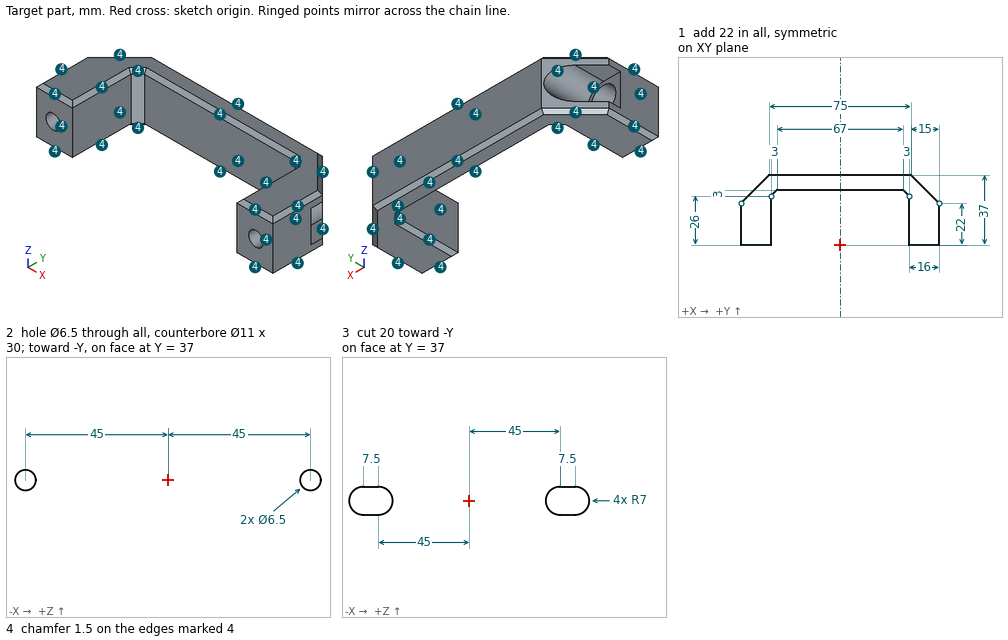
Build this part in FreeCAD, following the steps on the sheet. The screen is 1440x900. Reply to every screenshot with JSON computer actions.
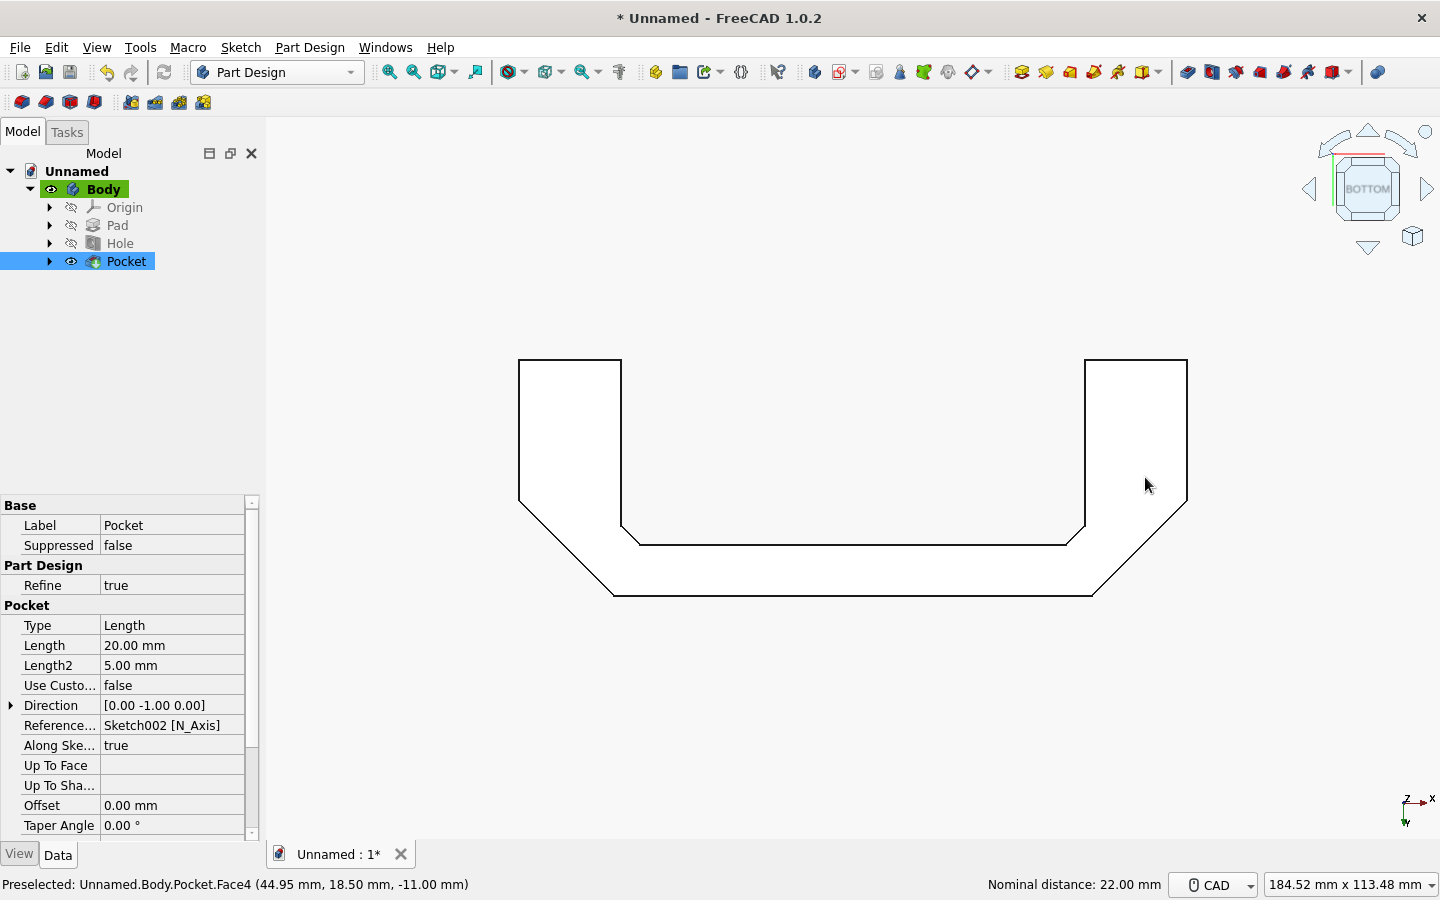
{"action": "left_click", "coordinate": [46, 102]}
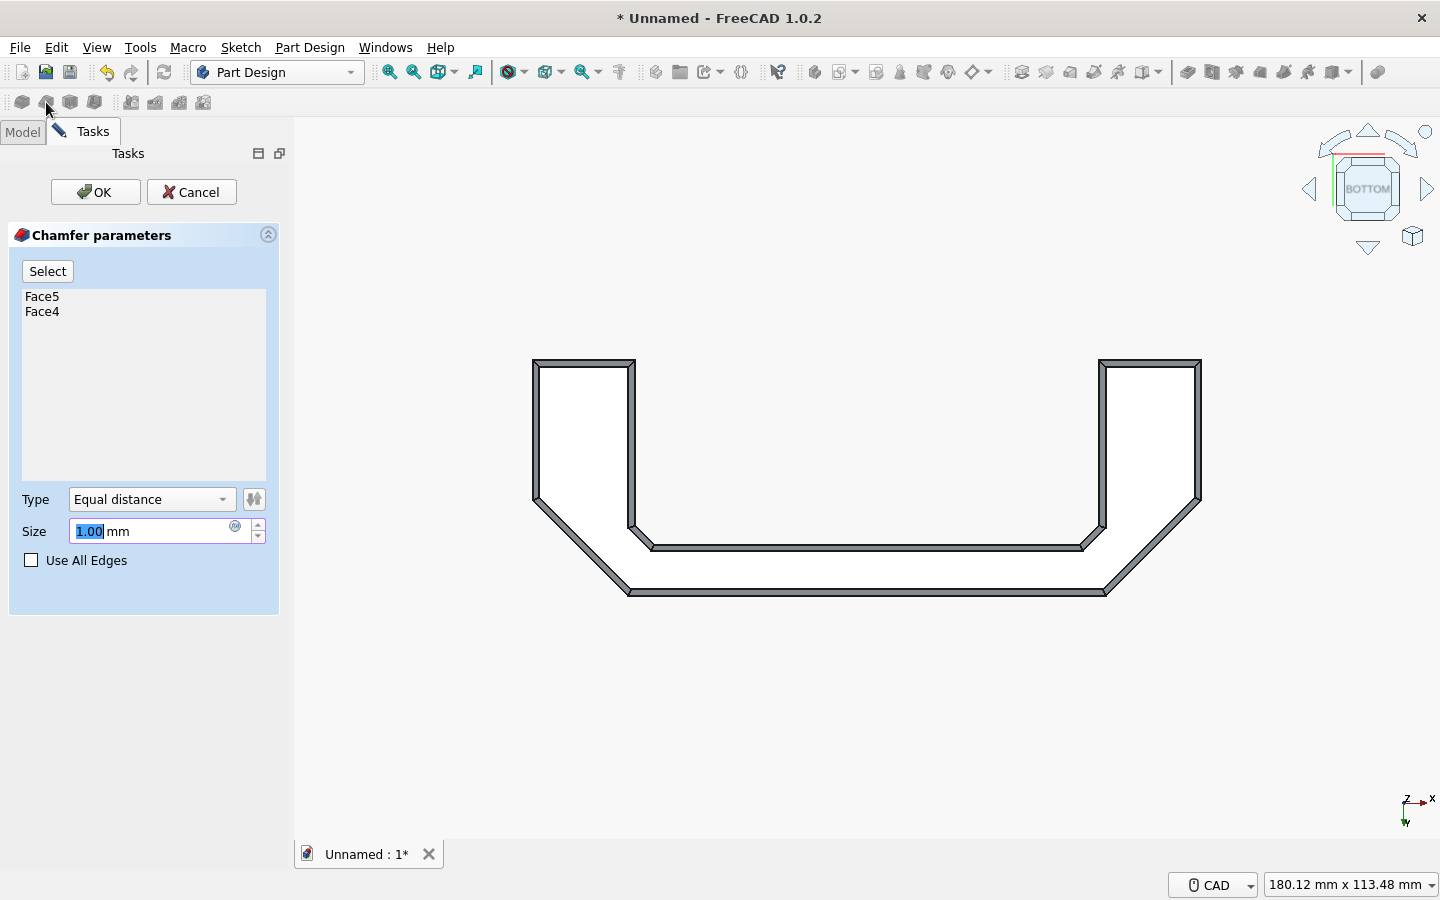
{"action": "type", "text": "1.5"}
{"action": "key", "text": "Tab"}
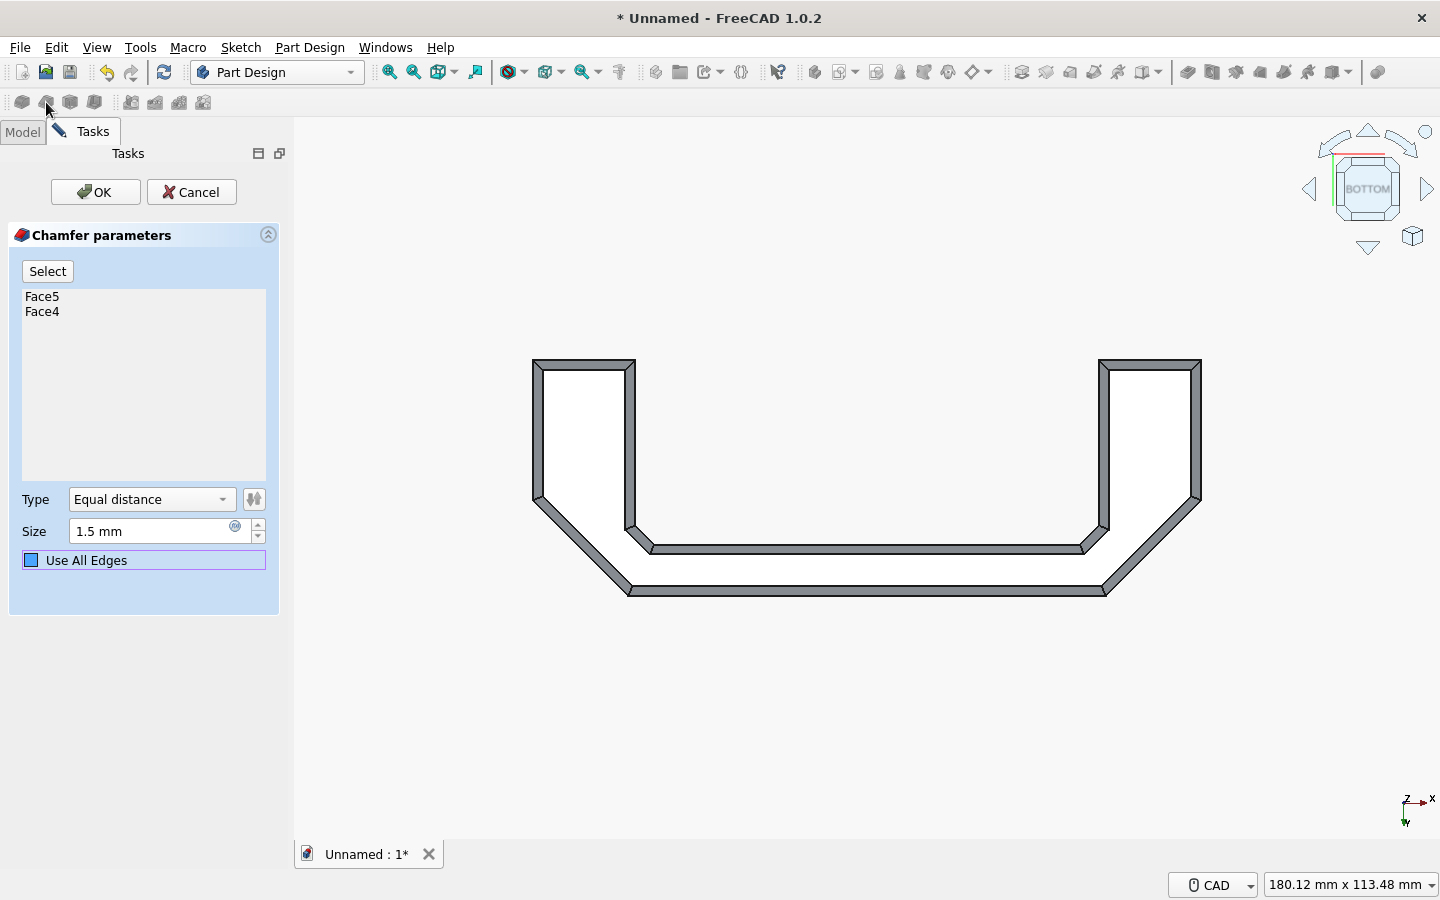
{"action": "left_click", "coordinate": [96, 192]}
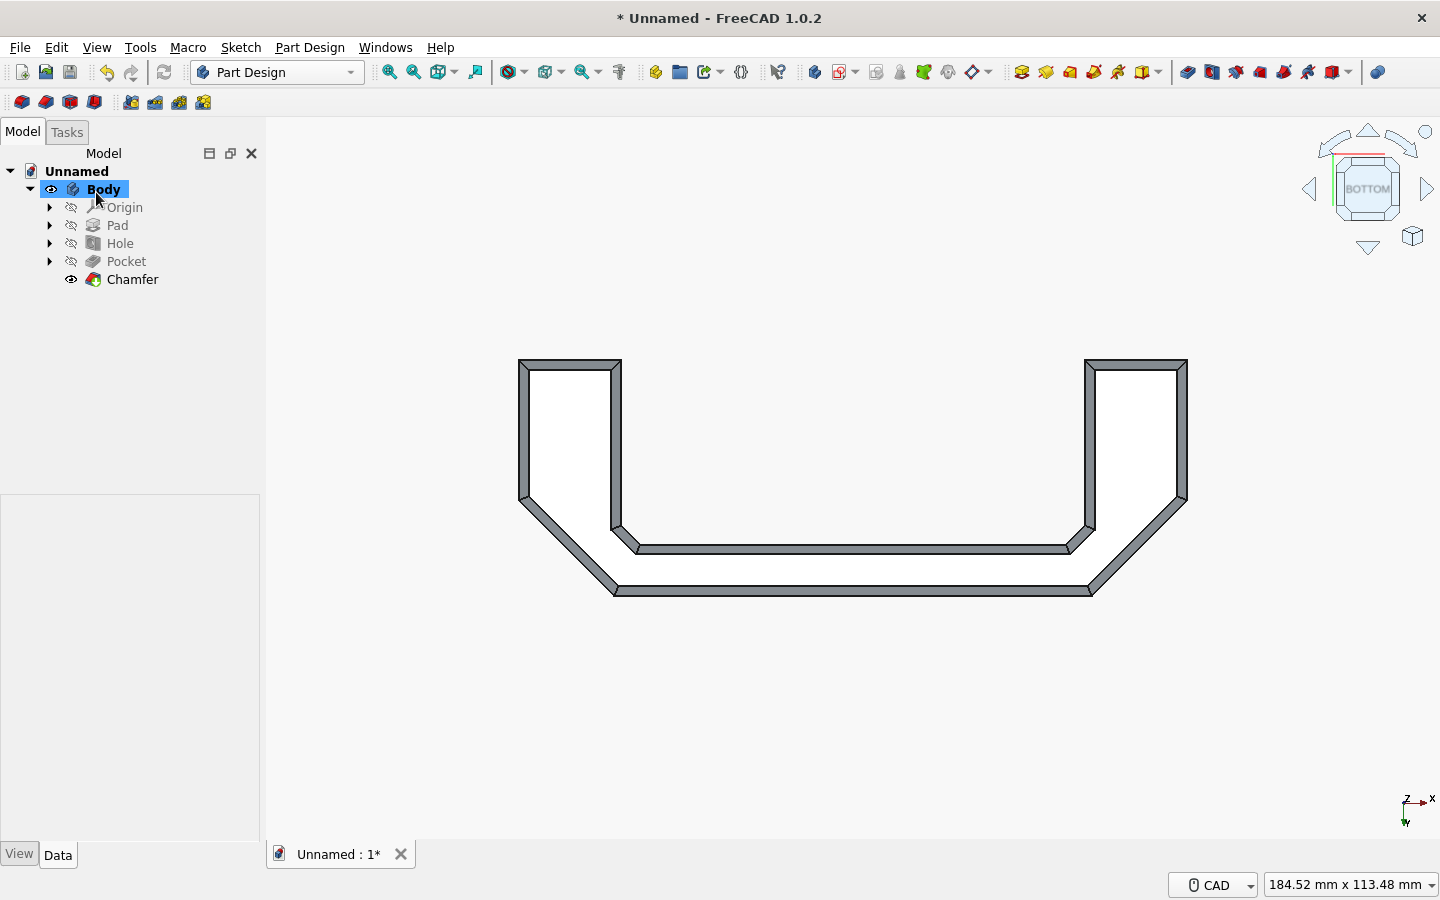
{"action": "key", "text": "0"}